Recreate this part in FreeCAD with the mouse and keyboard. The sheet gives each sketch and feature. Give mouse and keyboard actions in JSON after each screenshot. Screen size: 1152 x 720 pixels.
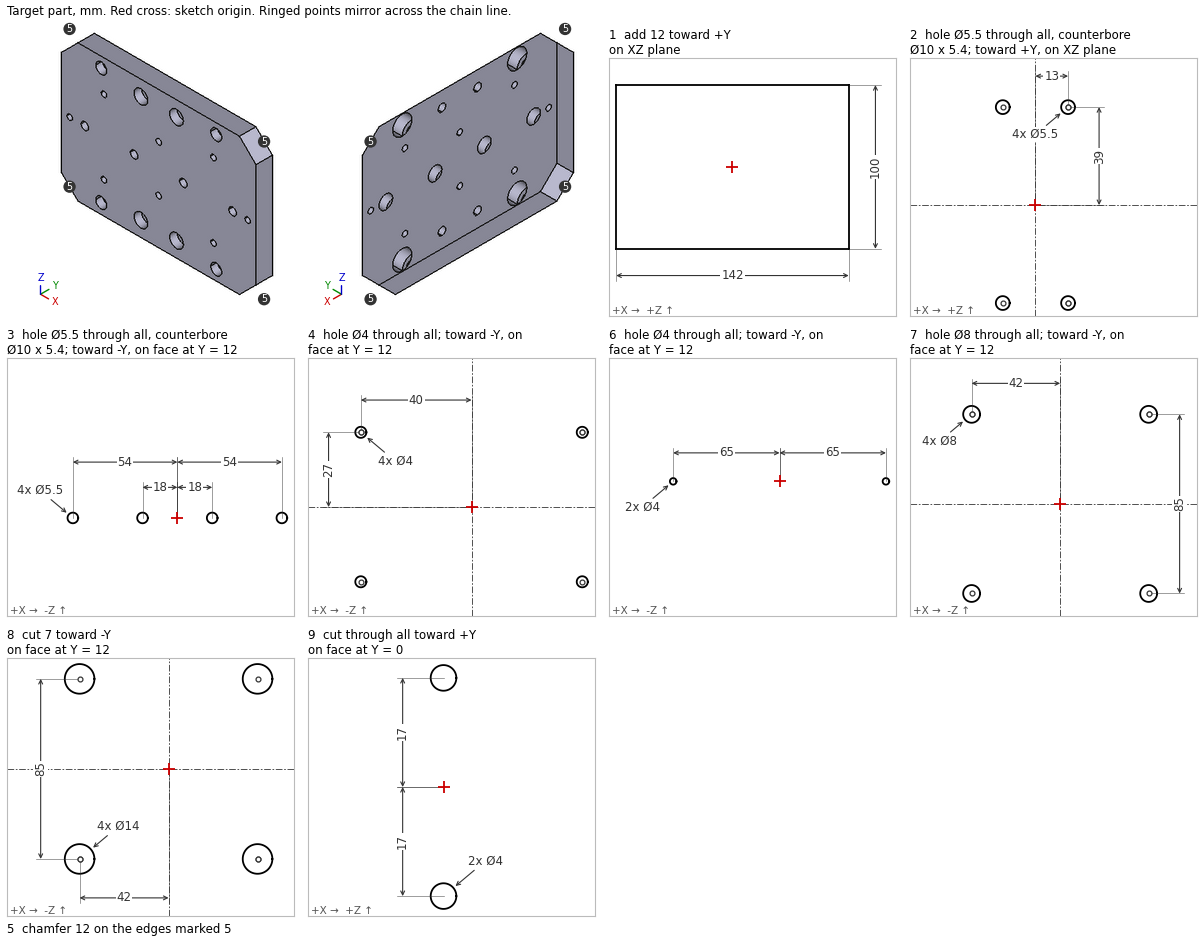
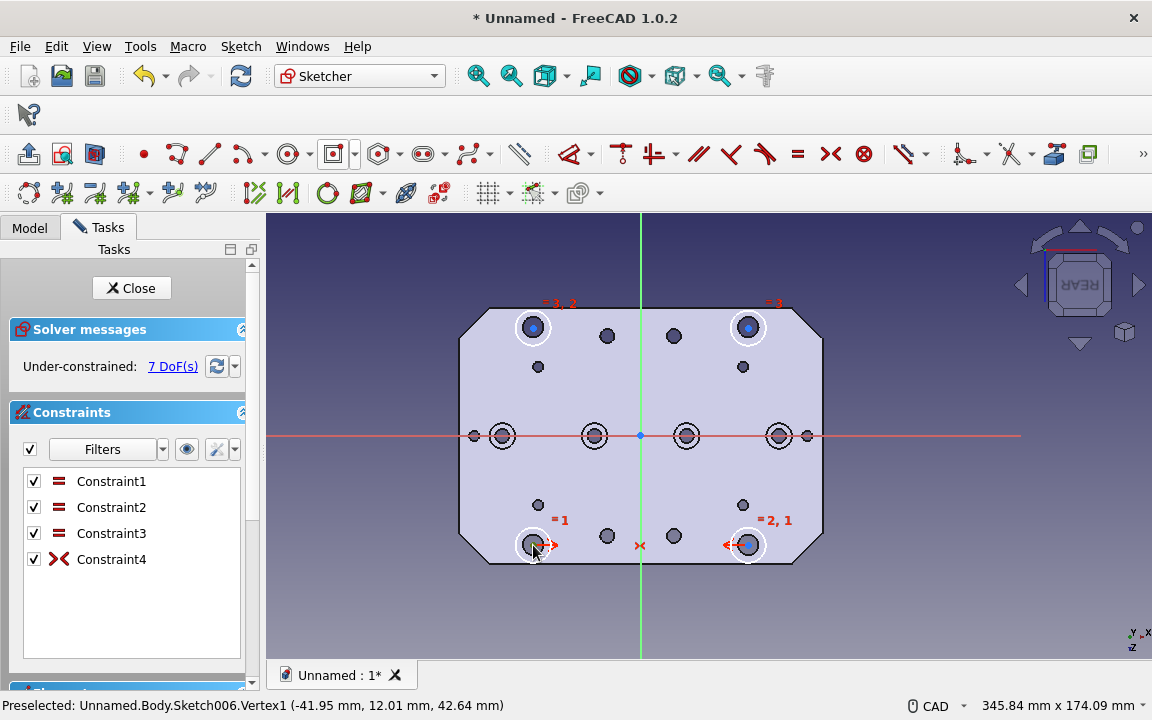
{"action": "left_click", "coordinate": [533, 328]}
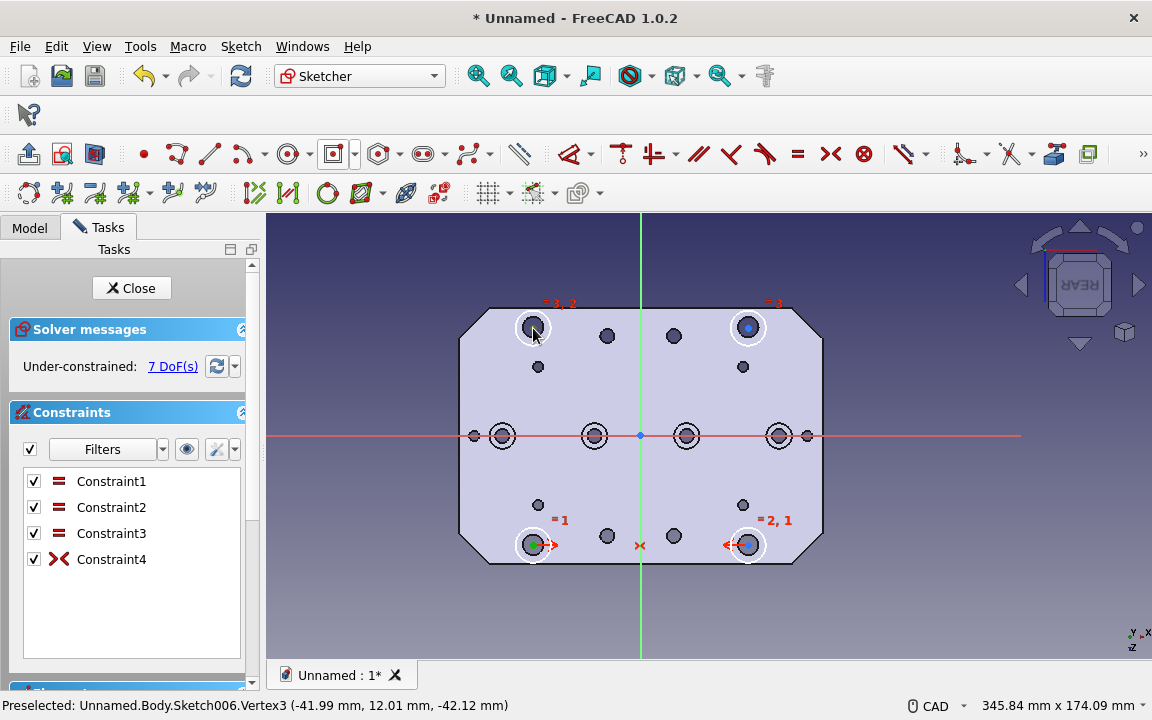
{"action": "left_click", "coordinate": [344, 436]}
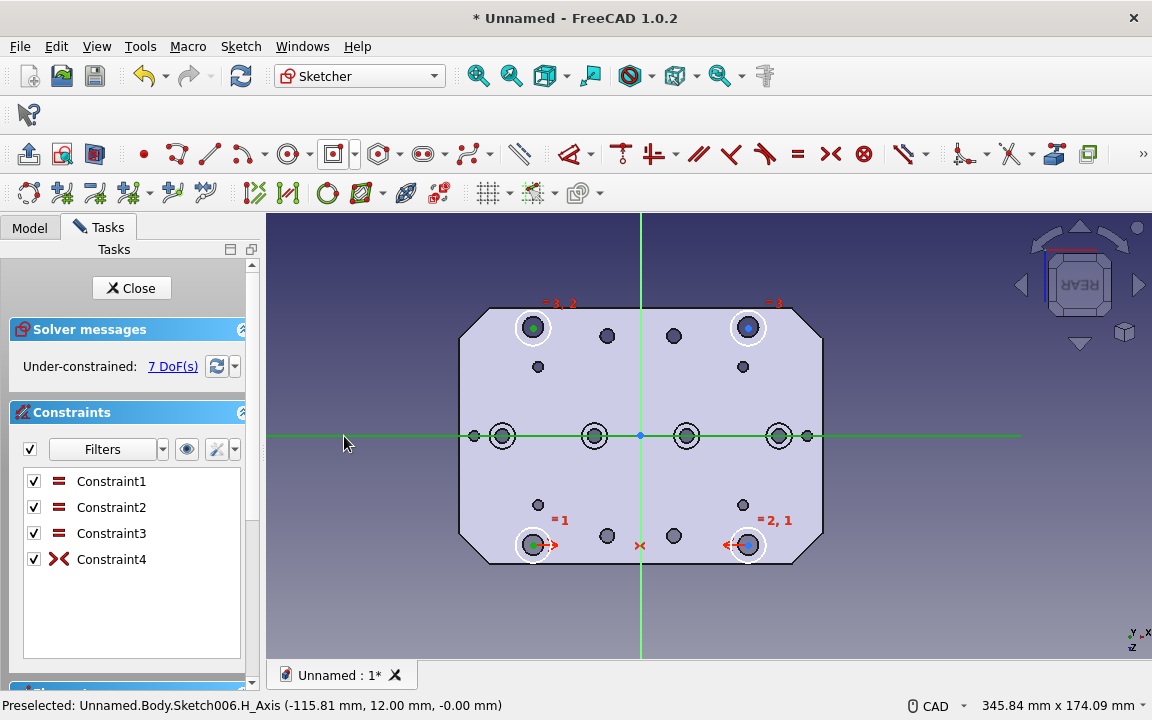
{"action": "left_click", "coordinate": [831, 154]}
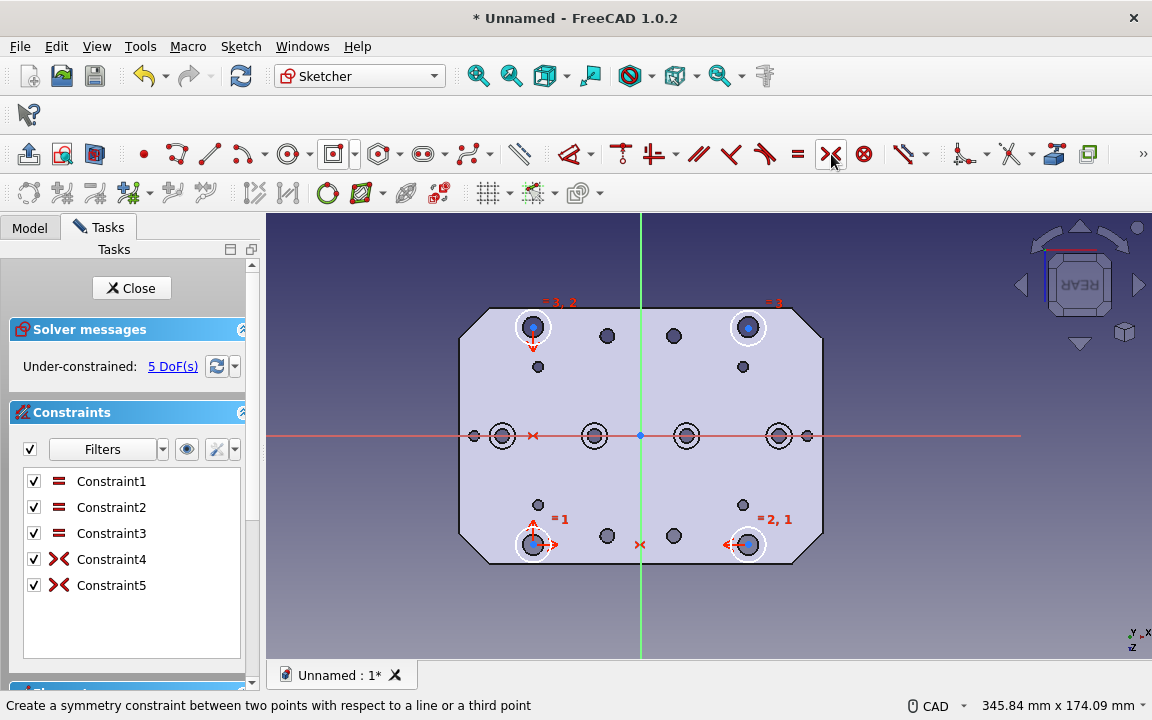
{"action": "left_click", "coordinate": [748, 545]}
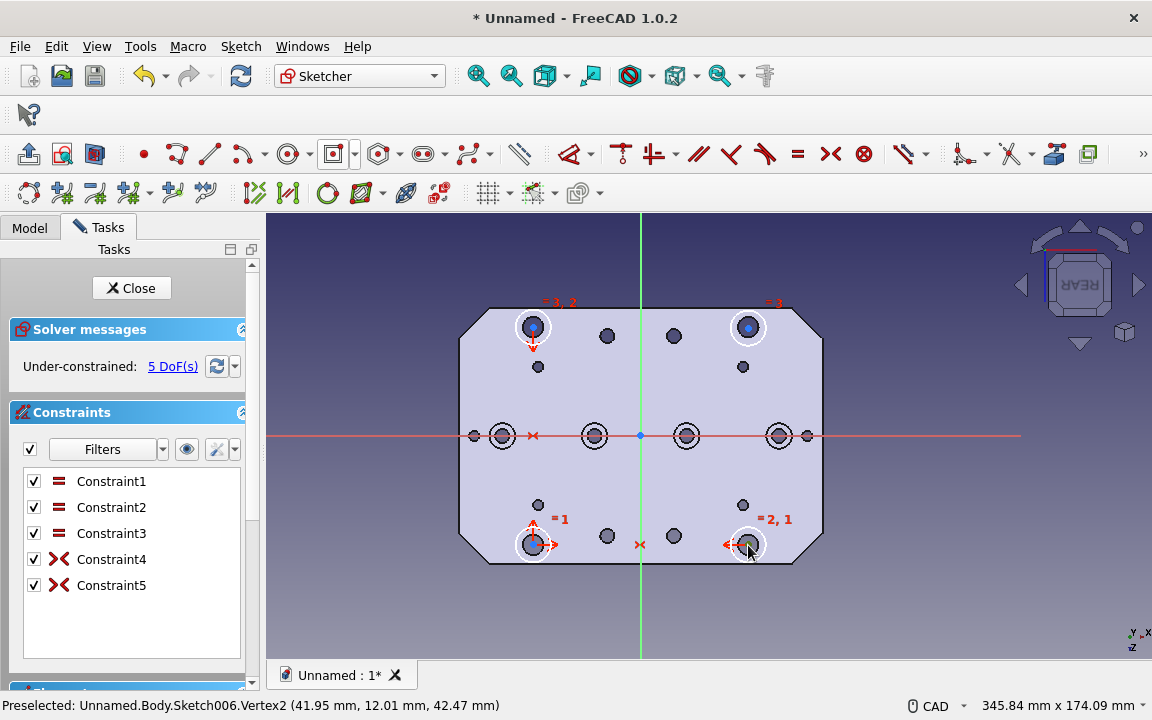
{"action": "left_click", "coordinate": [748, 328]}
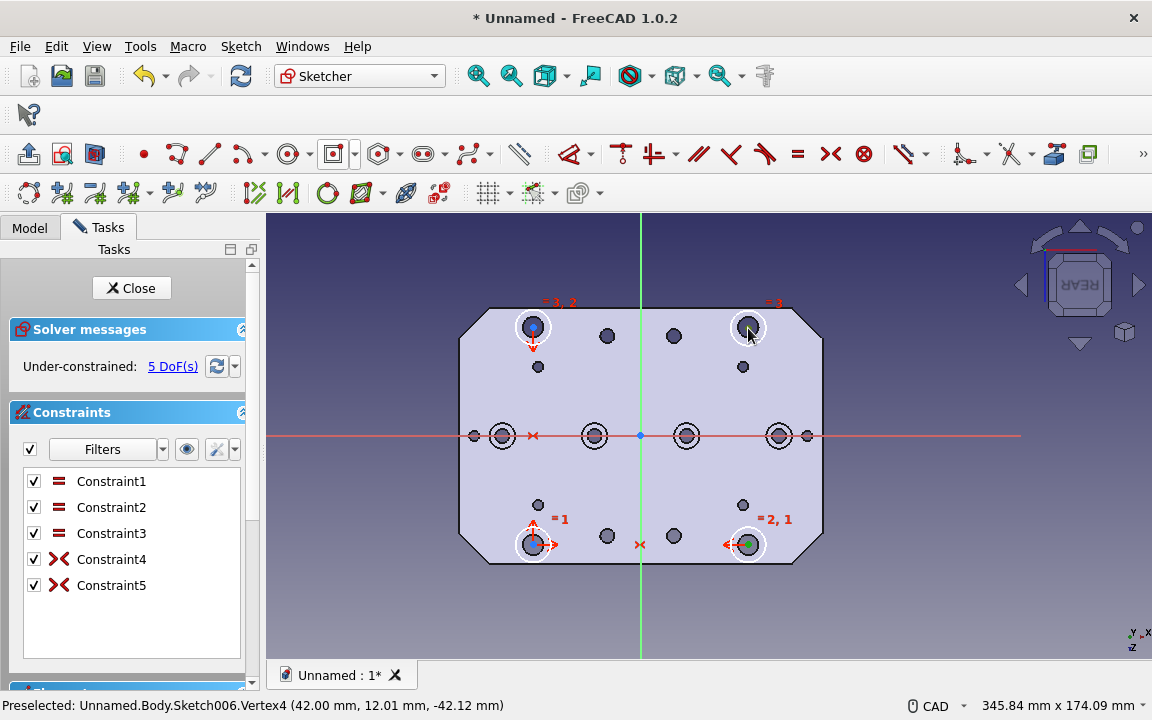
{"action": "left_click", "coordinate": [344, 436]}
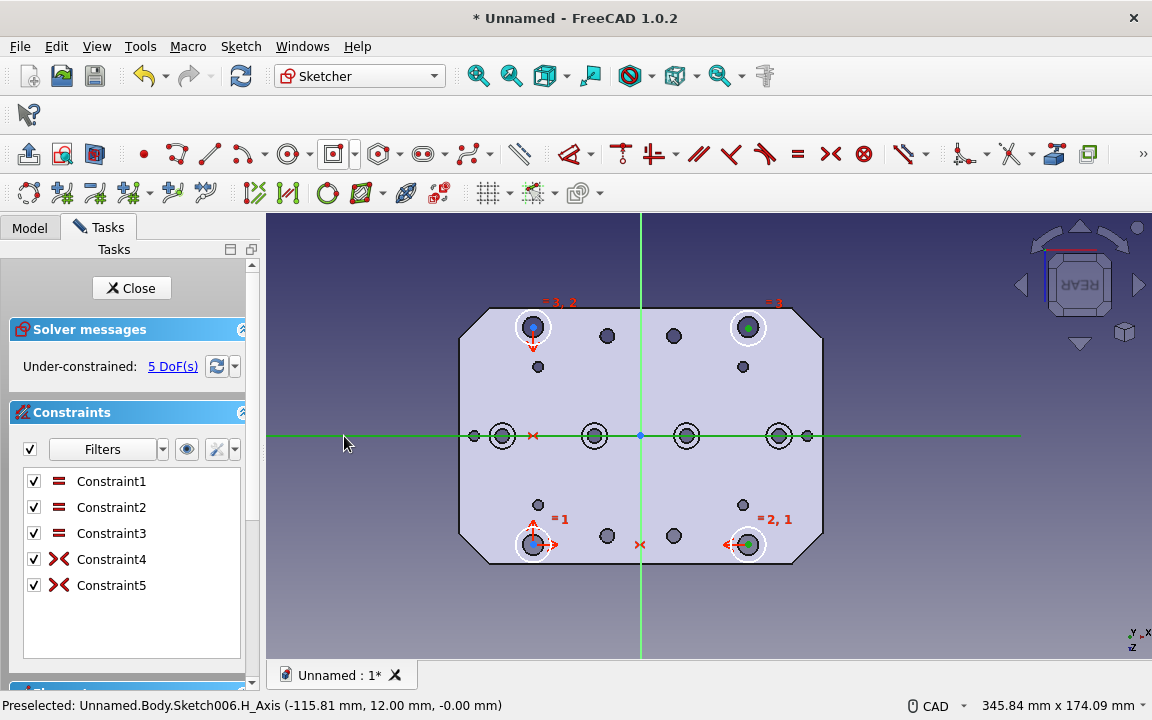
{"action": "left_click", "coordinate": [831, 154]}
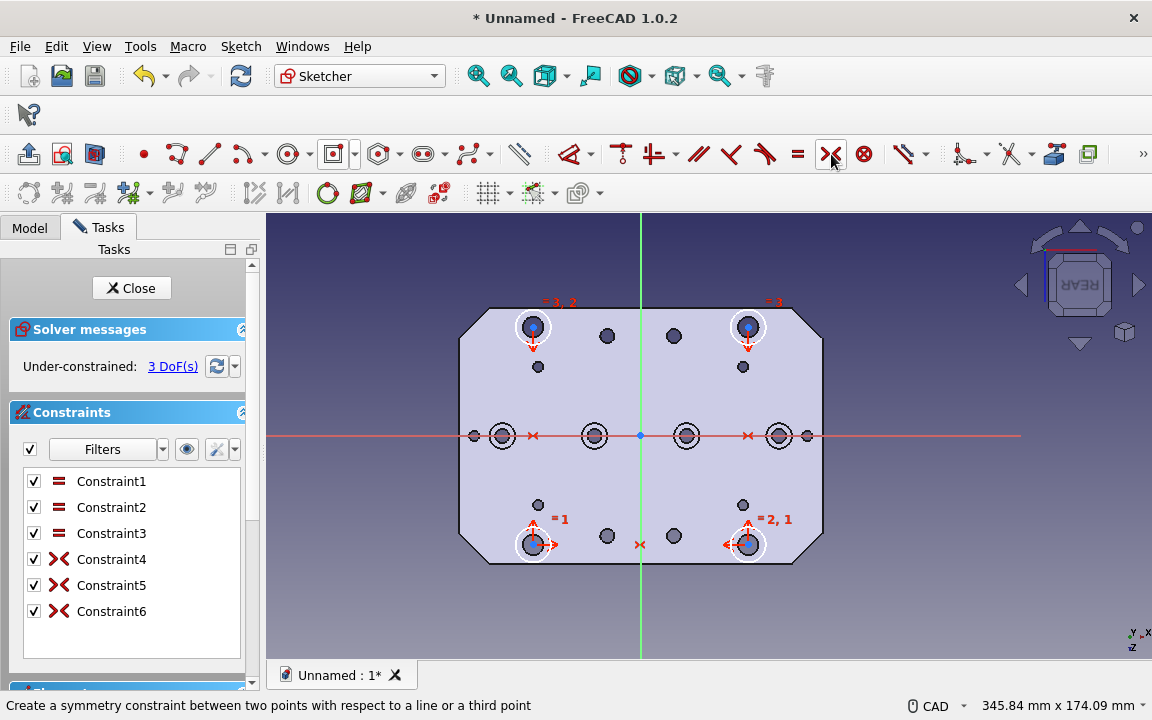
{"action": "left_click", "coordinate": [568, 154]}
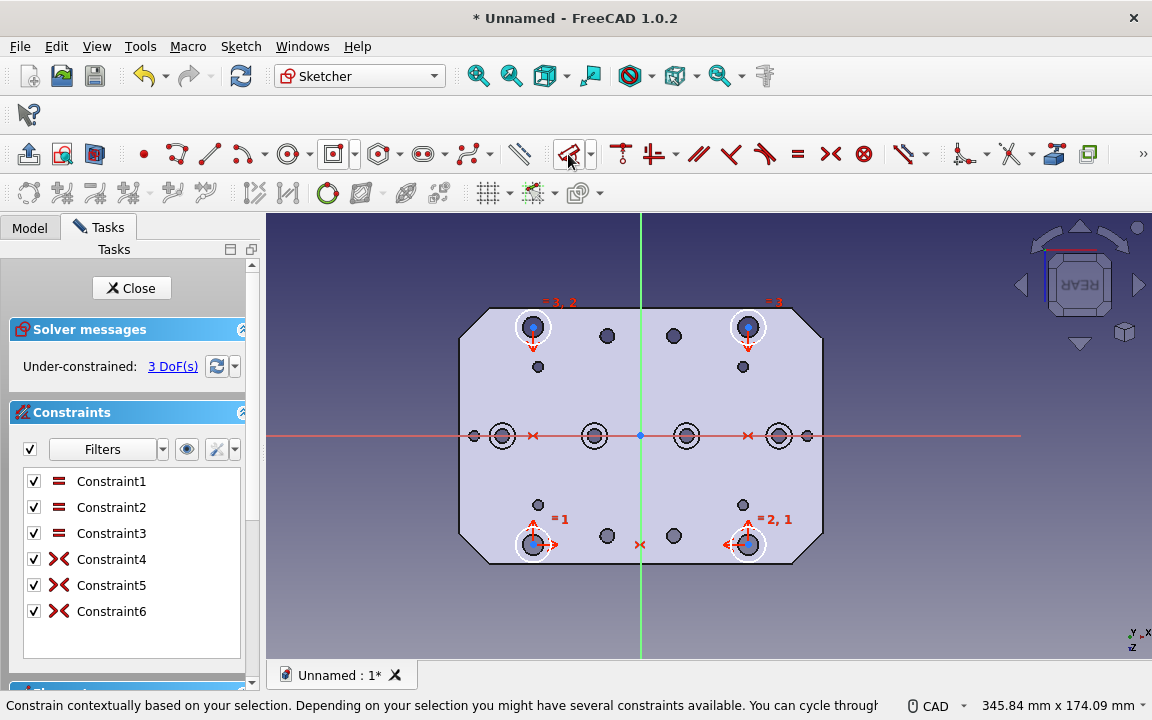
{"action": "left_click", "coordinate": [546, 532]}
{"action": "left_click", "coordinate": [569, 509]}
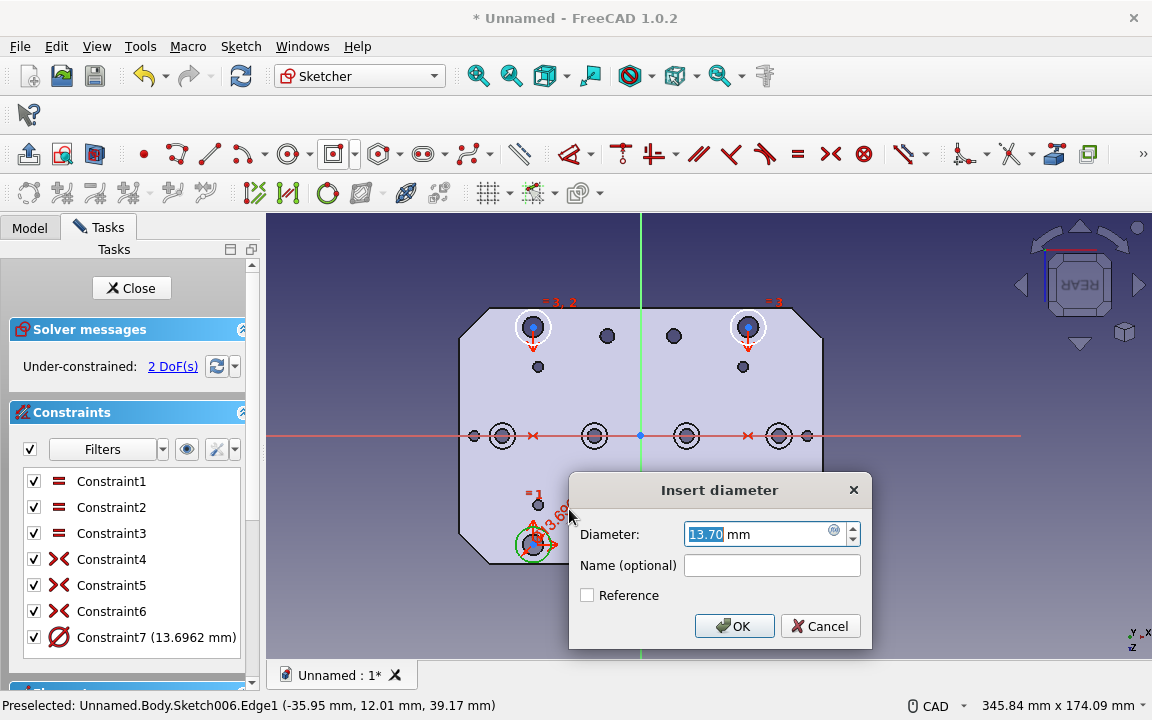
{"action": "type", "text": "14"}
{"action": "key", "text": "Return"}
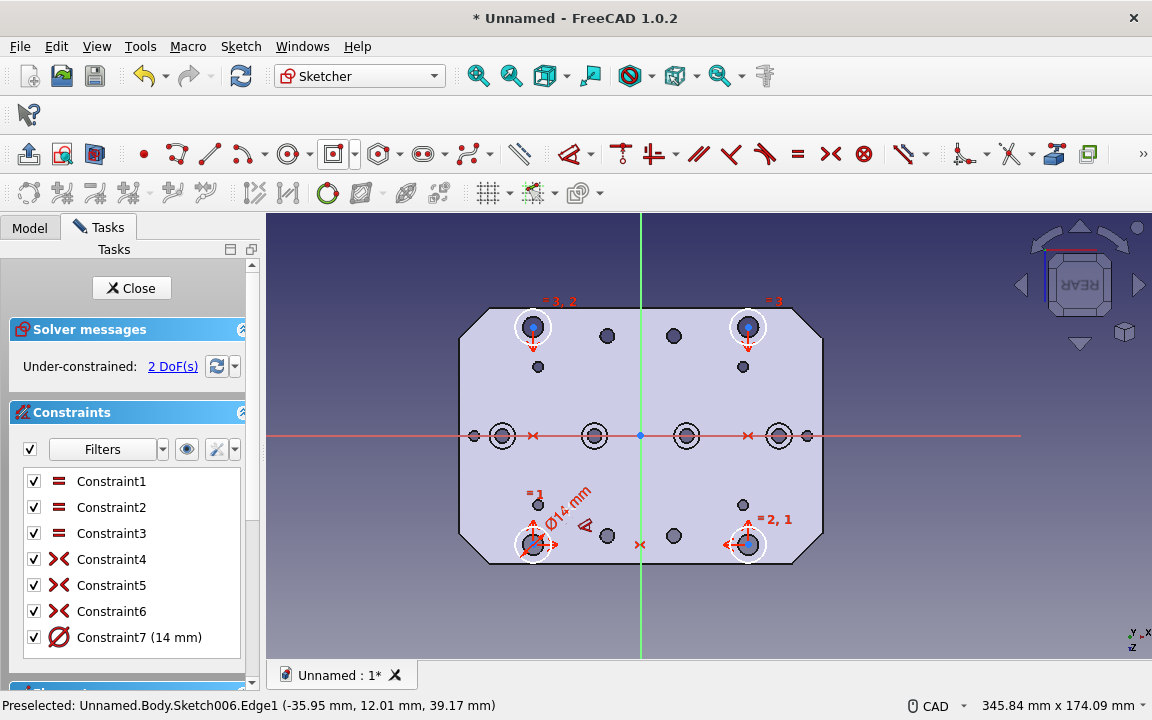
{"action": "left_click", "coordinate": [533, 545]}
{"action": "left_click", "coordinate": [587, 579]}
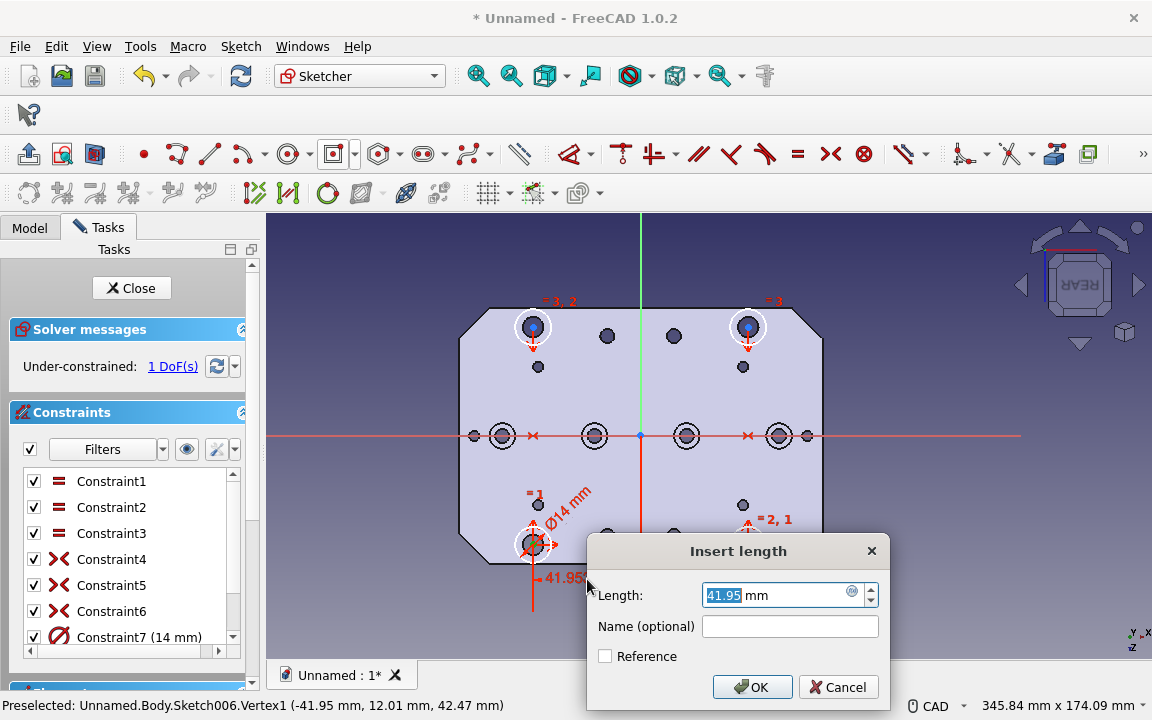
{"action": "type", "text": "42"}
{"action": "key", "text": "Return"}